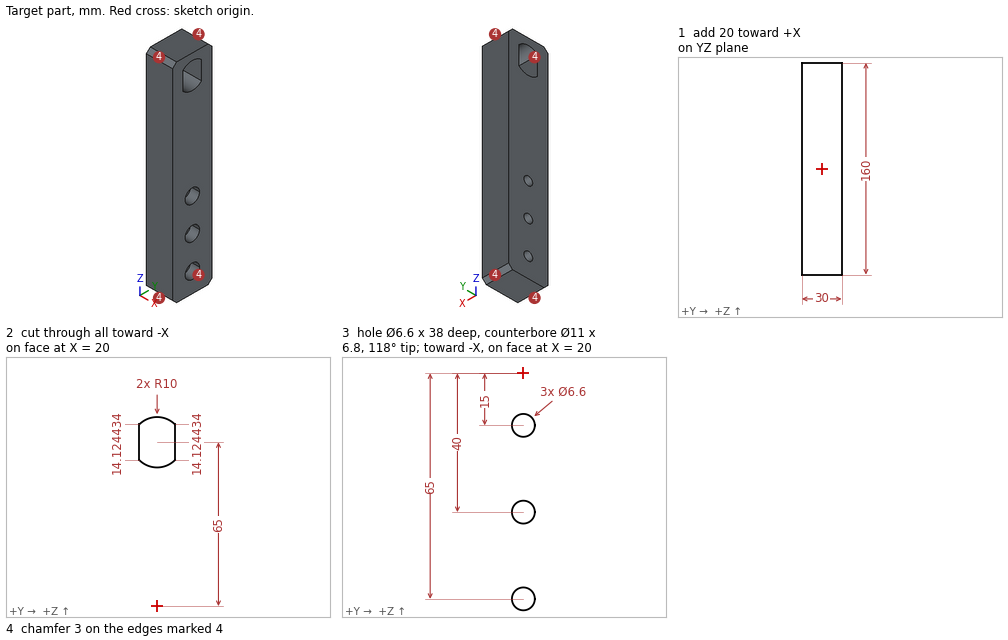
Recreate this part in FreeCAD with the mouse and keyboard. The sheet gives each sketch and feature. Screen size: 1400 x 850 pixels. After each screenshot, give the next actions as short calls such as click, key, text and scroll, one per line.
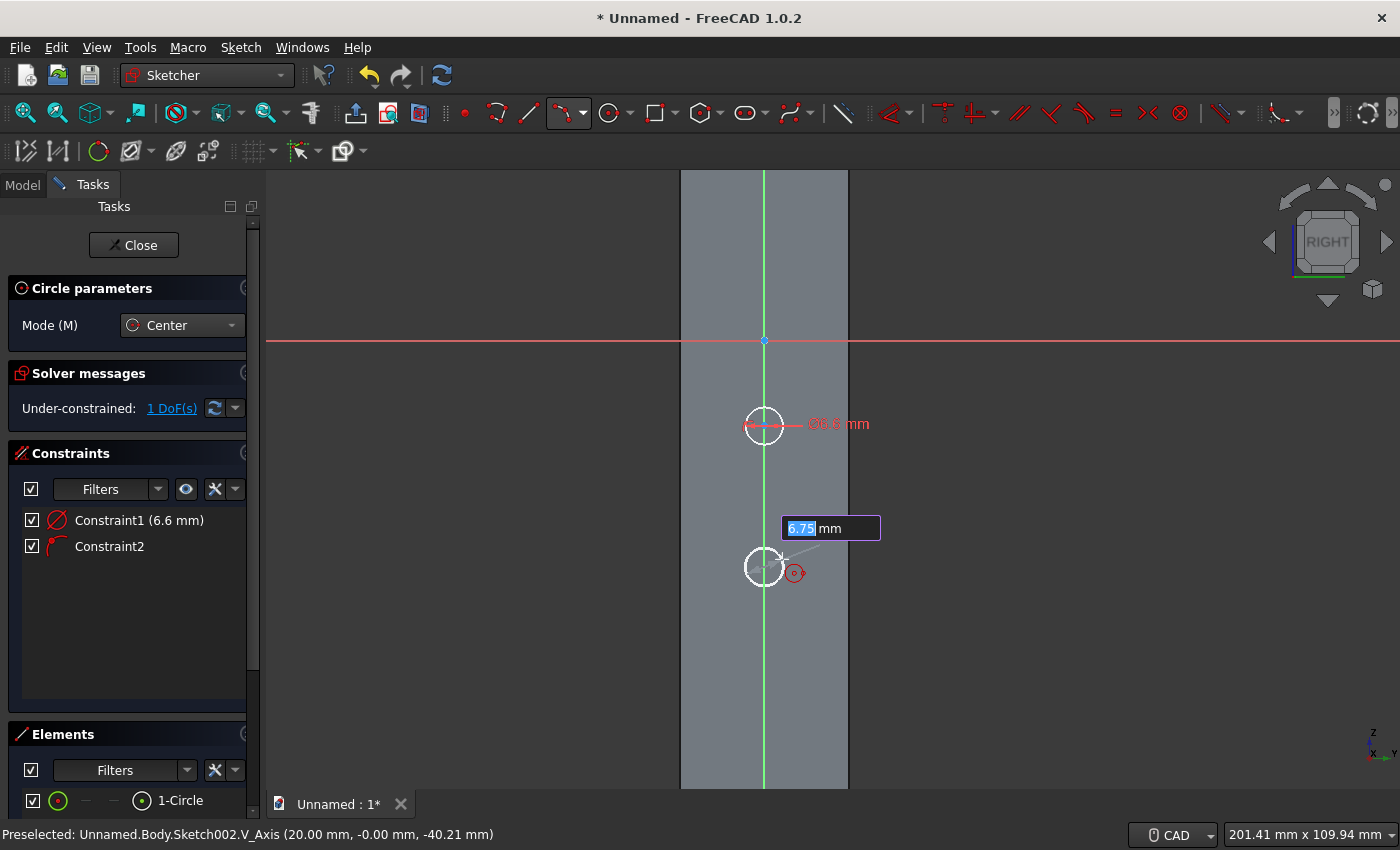
text(6.6)
key(Return)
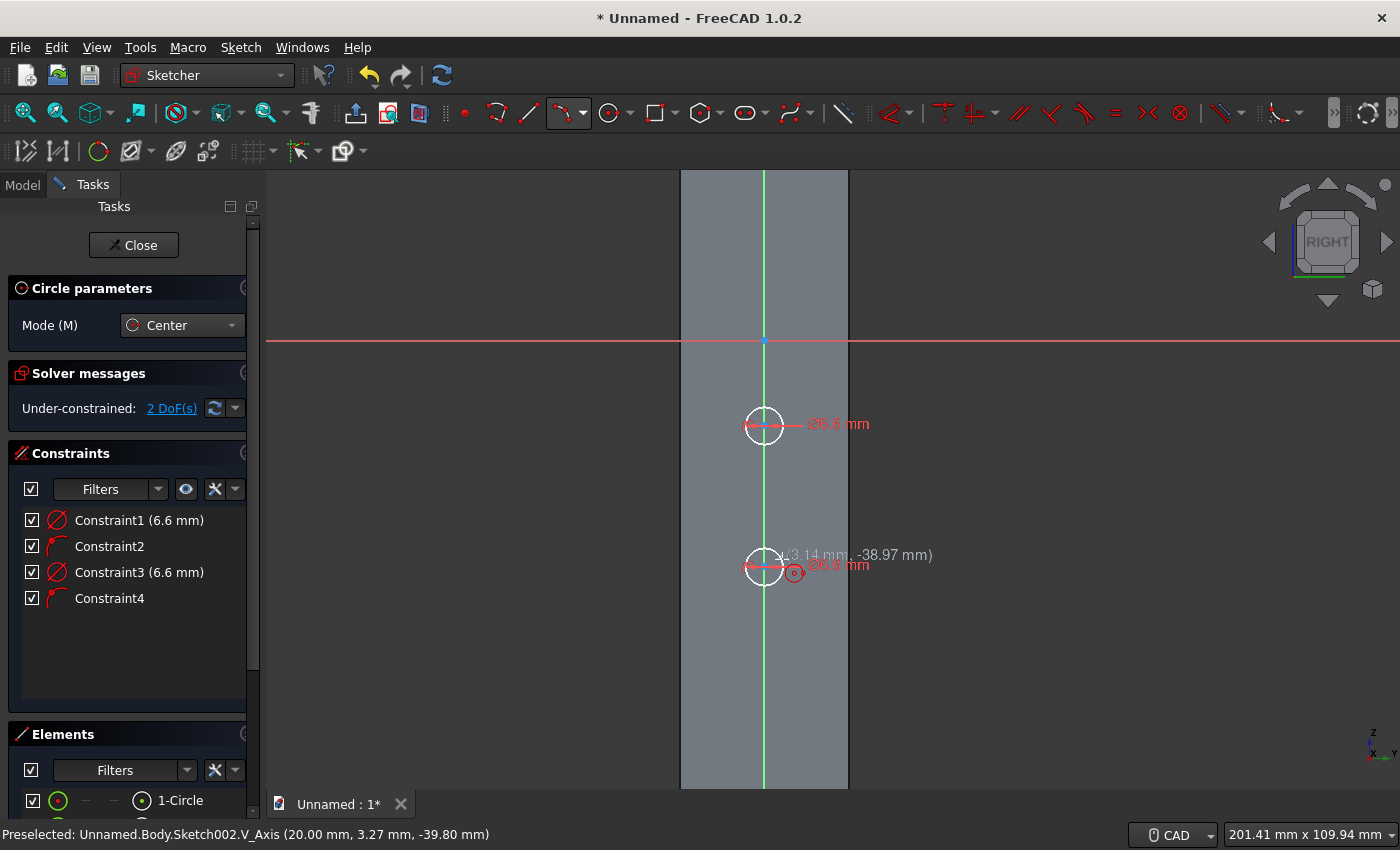
click(764, 707)
move(782, 700)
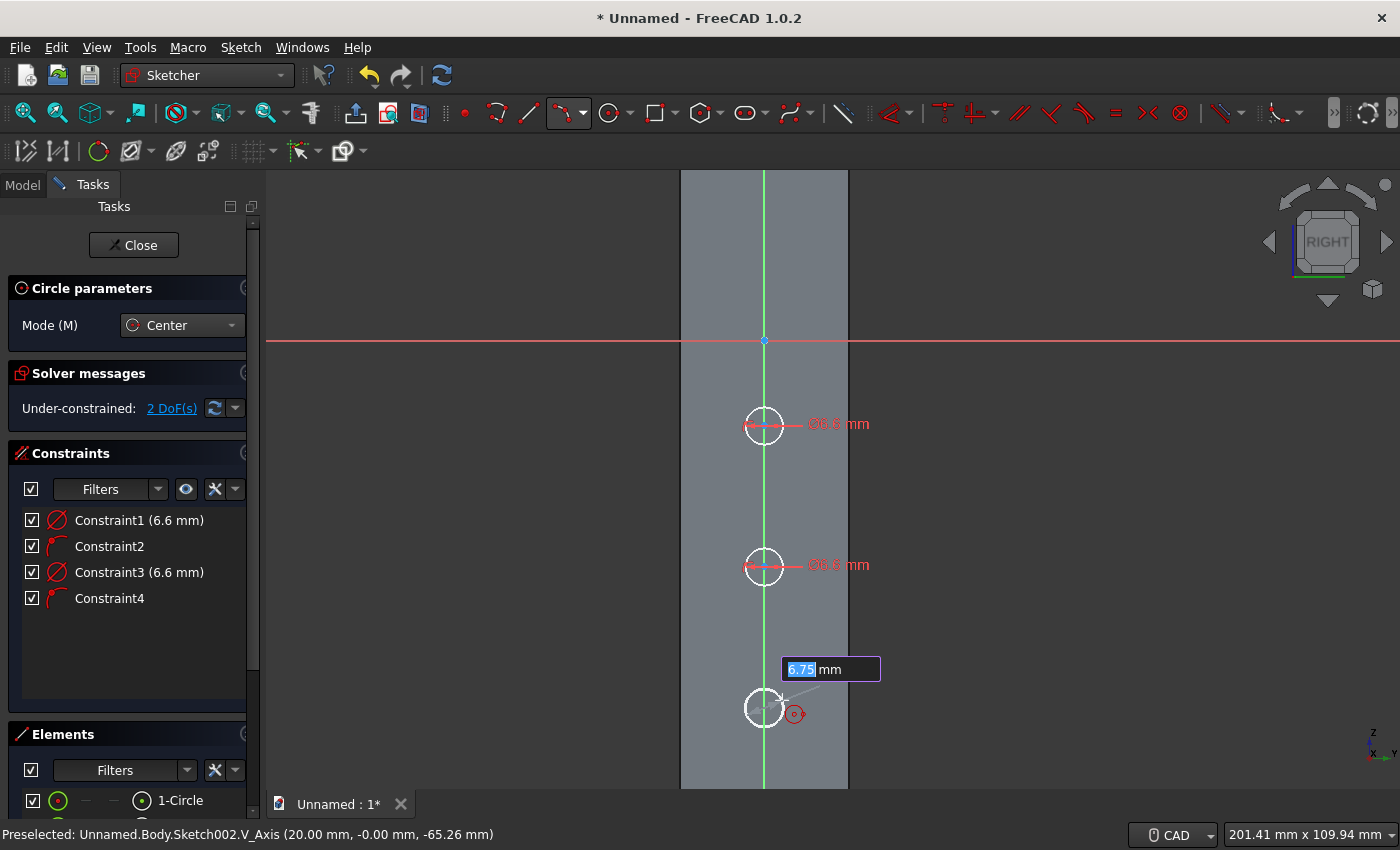
text(6.6)
key(Return)
key(Escape)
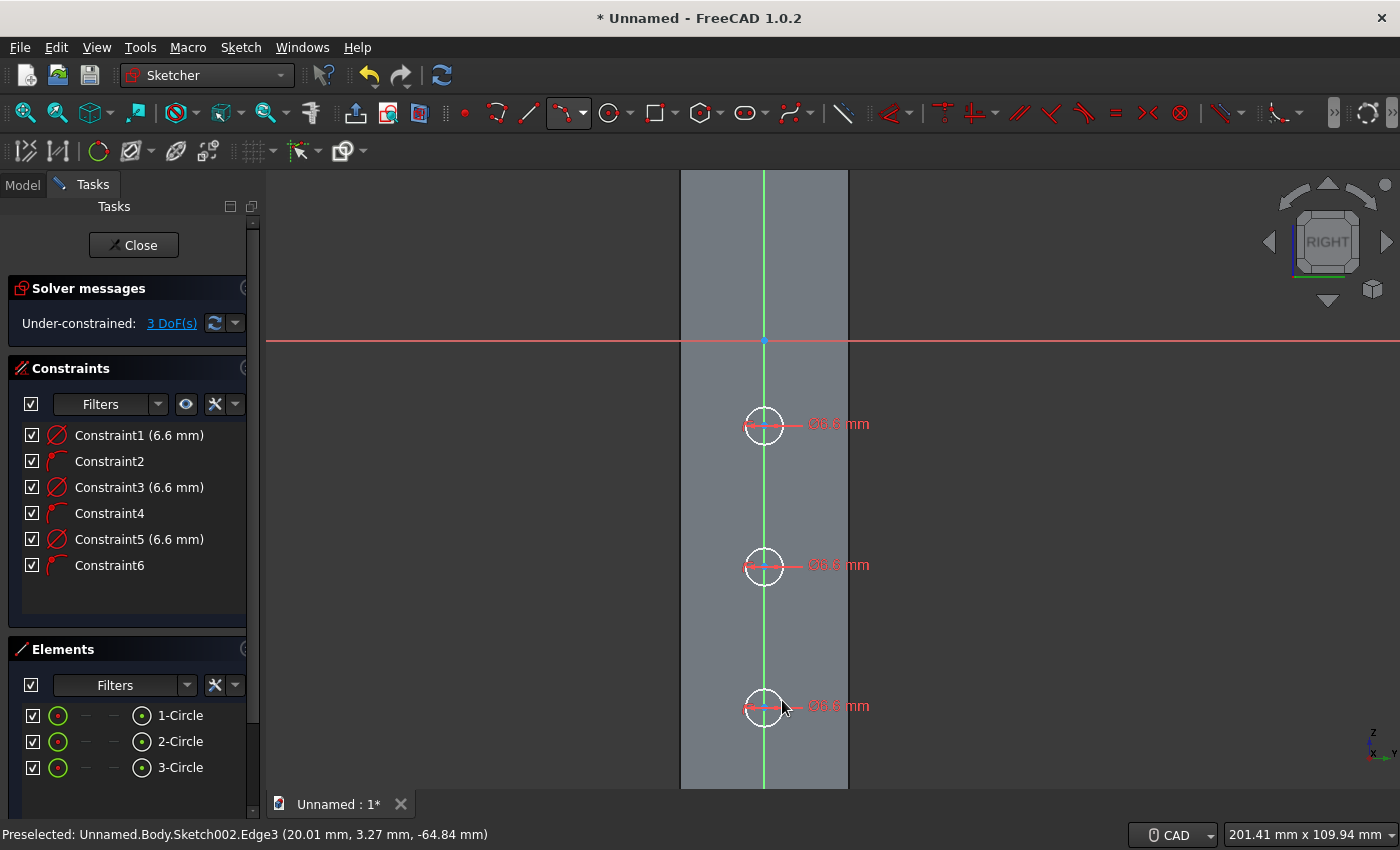
key(d)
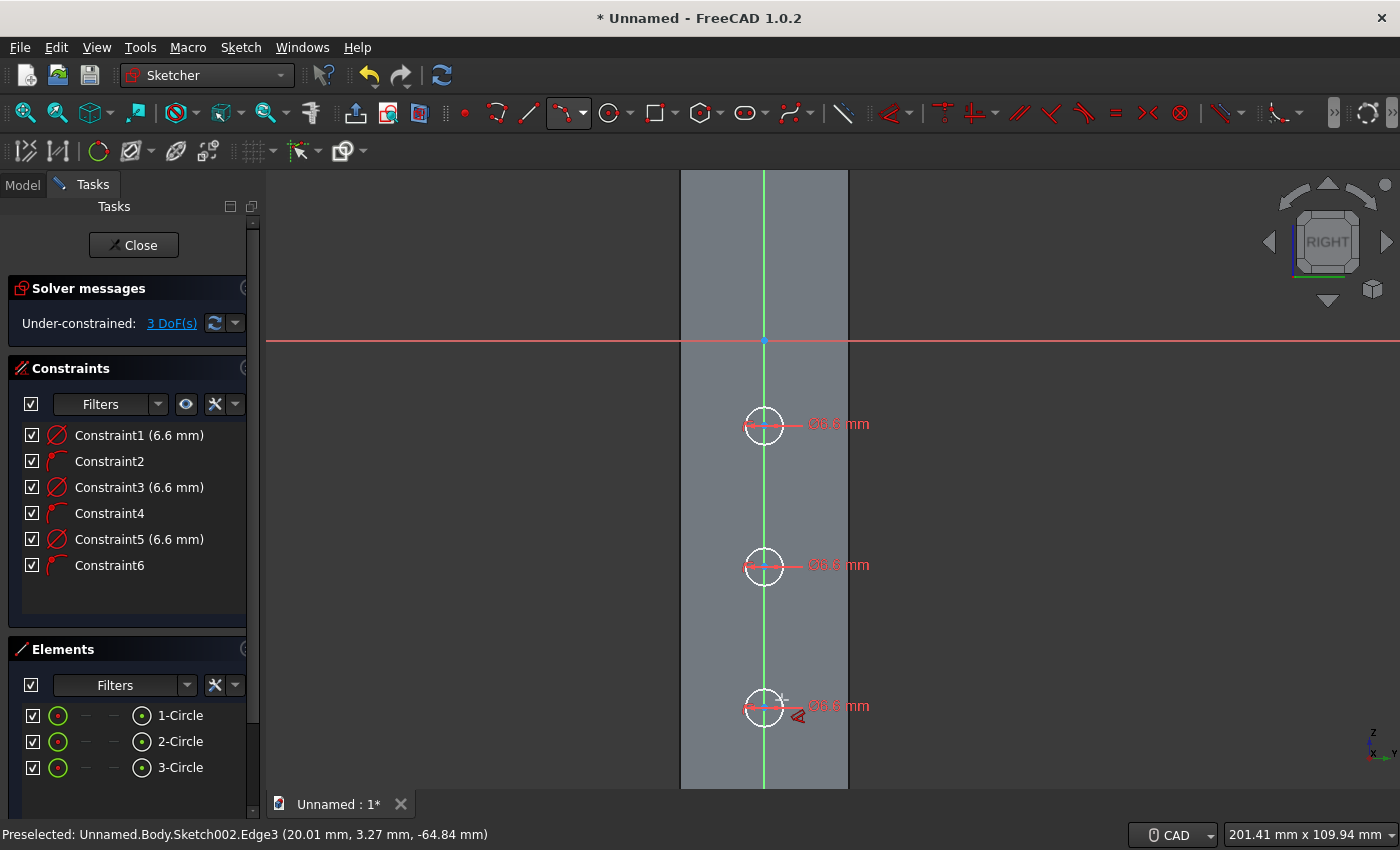
click(764, 426)
click(798, 383)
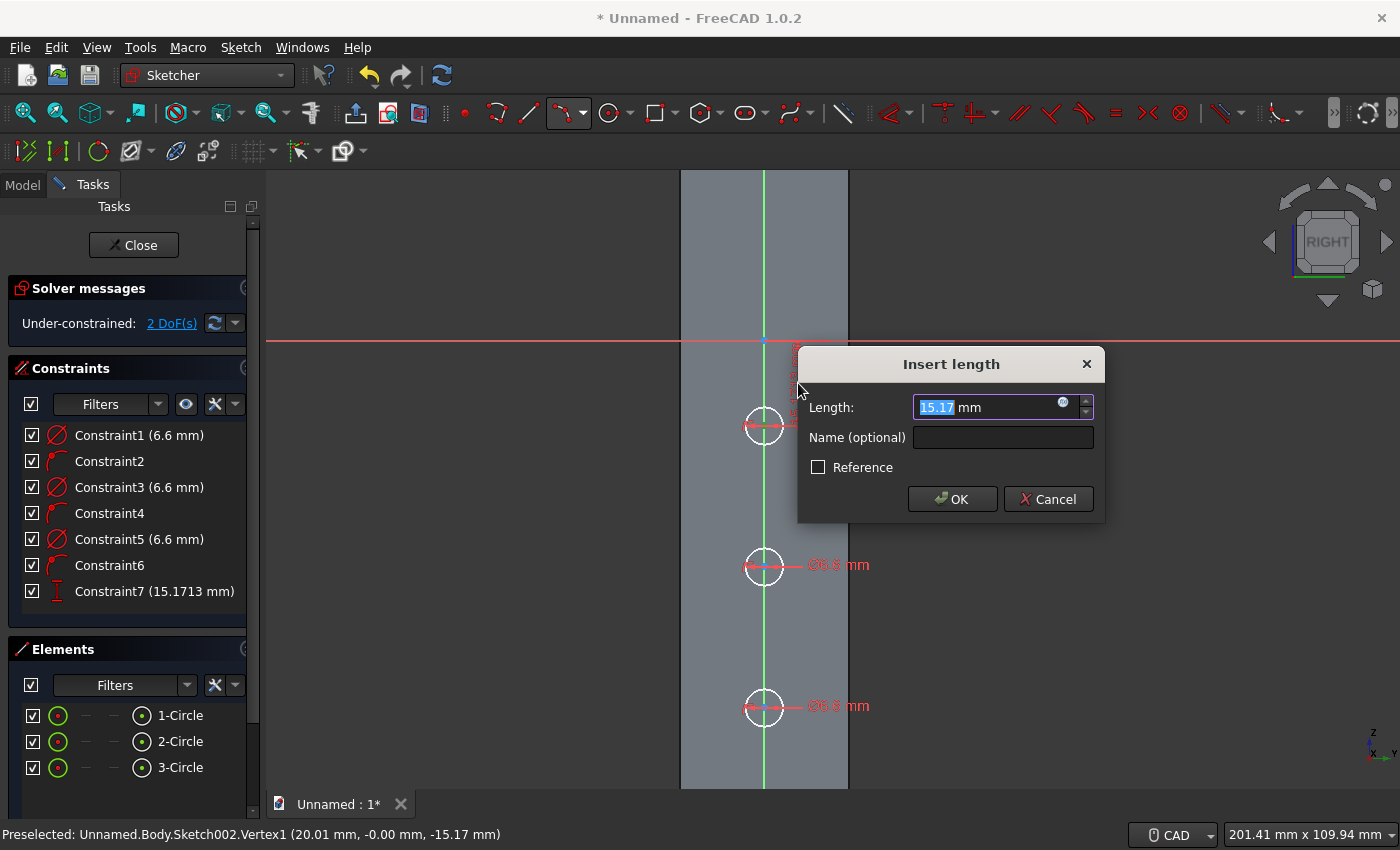
text(15)
key(Return)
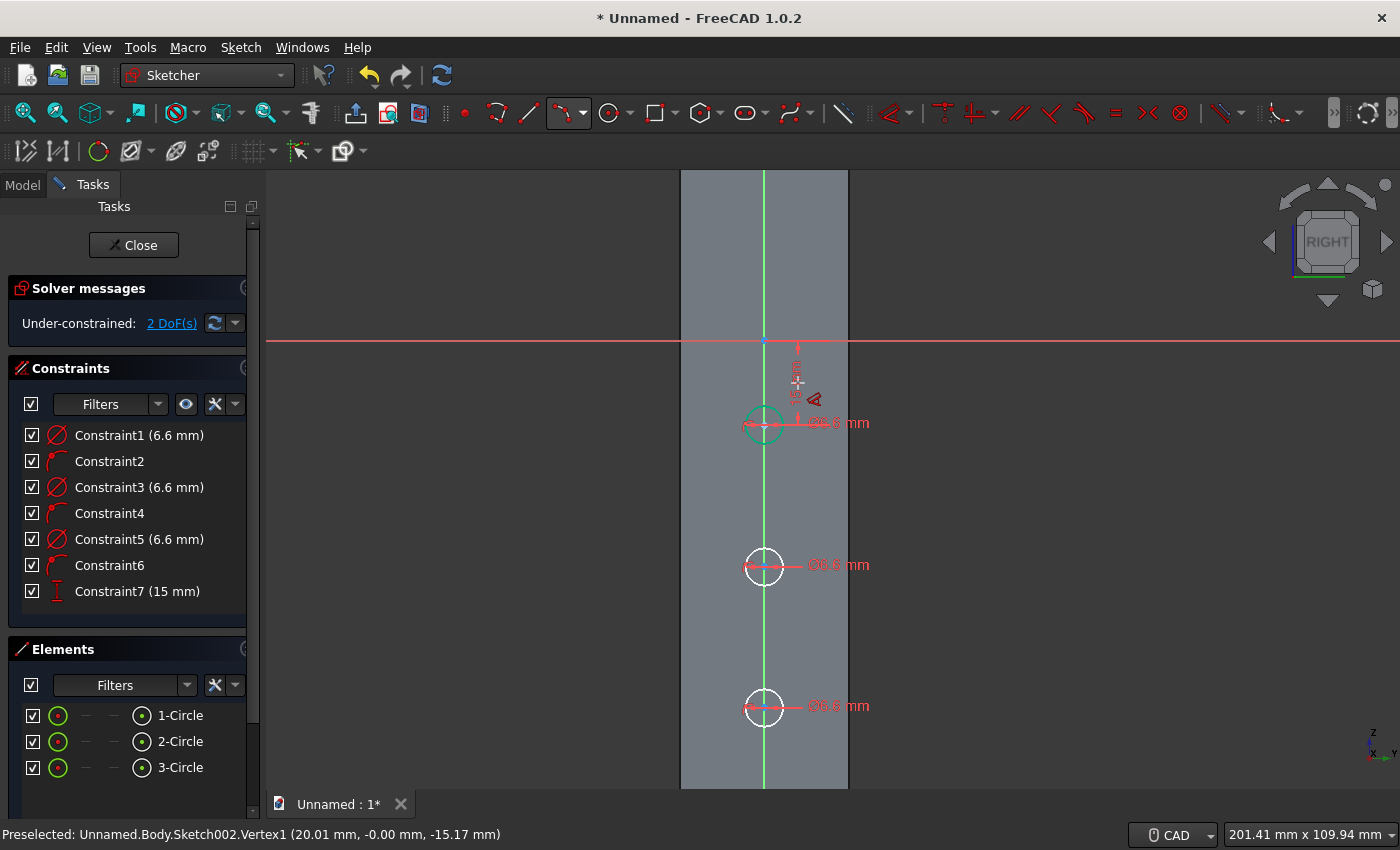
click(764, 567)
click(798, 454)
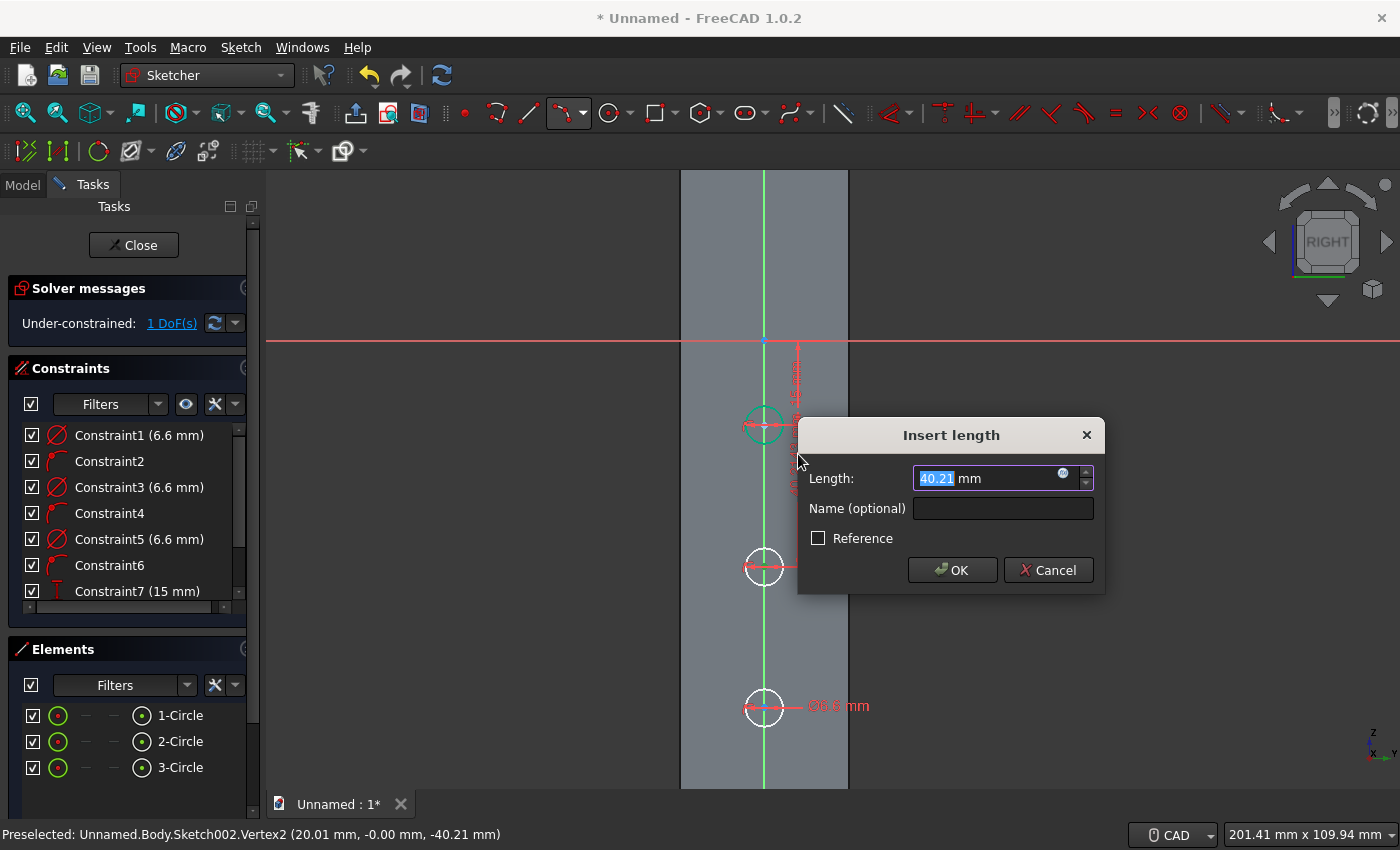
text(40)
key(Return)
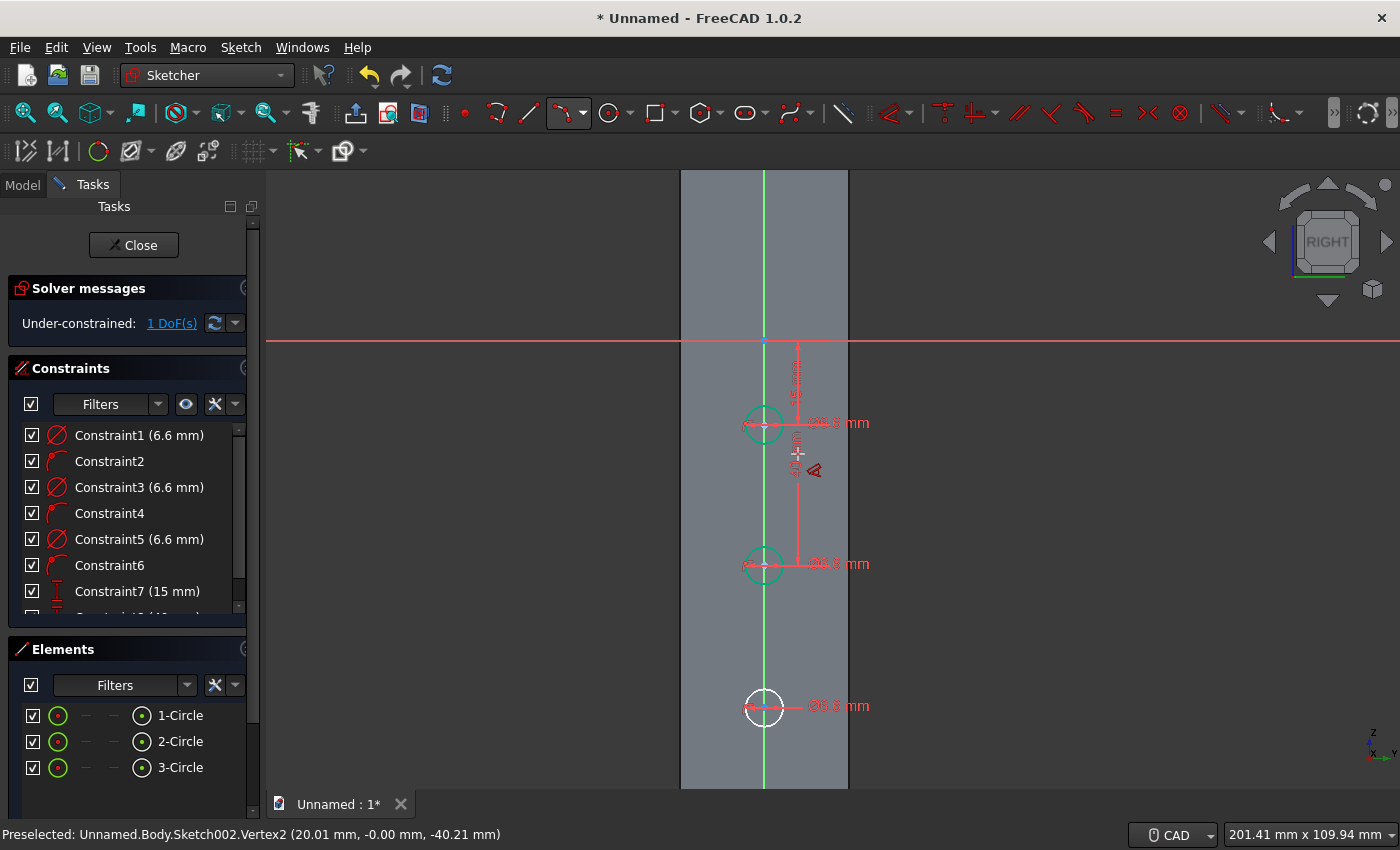
click(764, 708)
click(798, 524)